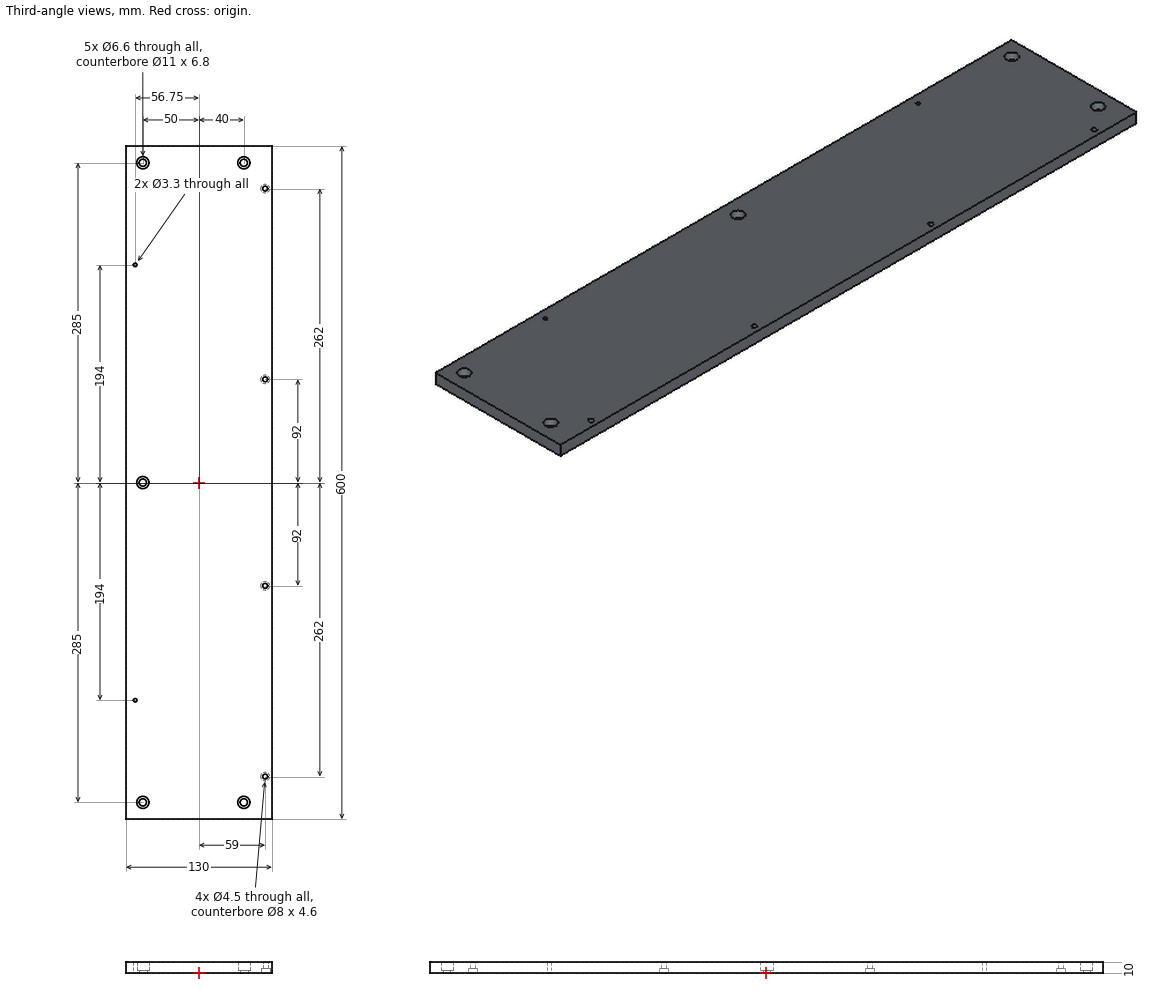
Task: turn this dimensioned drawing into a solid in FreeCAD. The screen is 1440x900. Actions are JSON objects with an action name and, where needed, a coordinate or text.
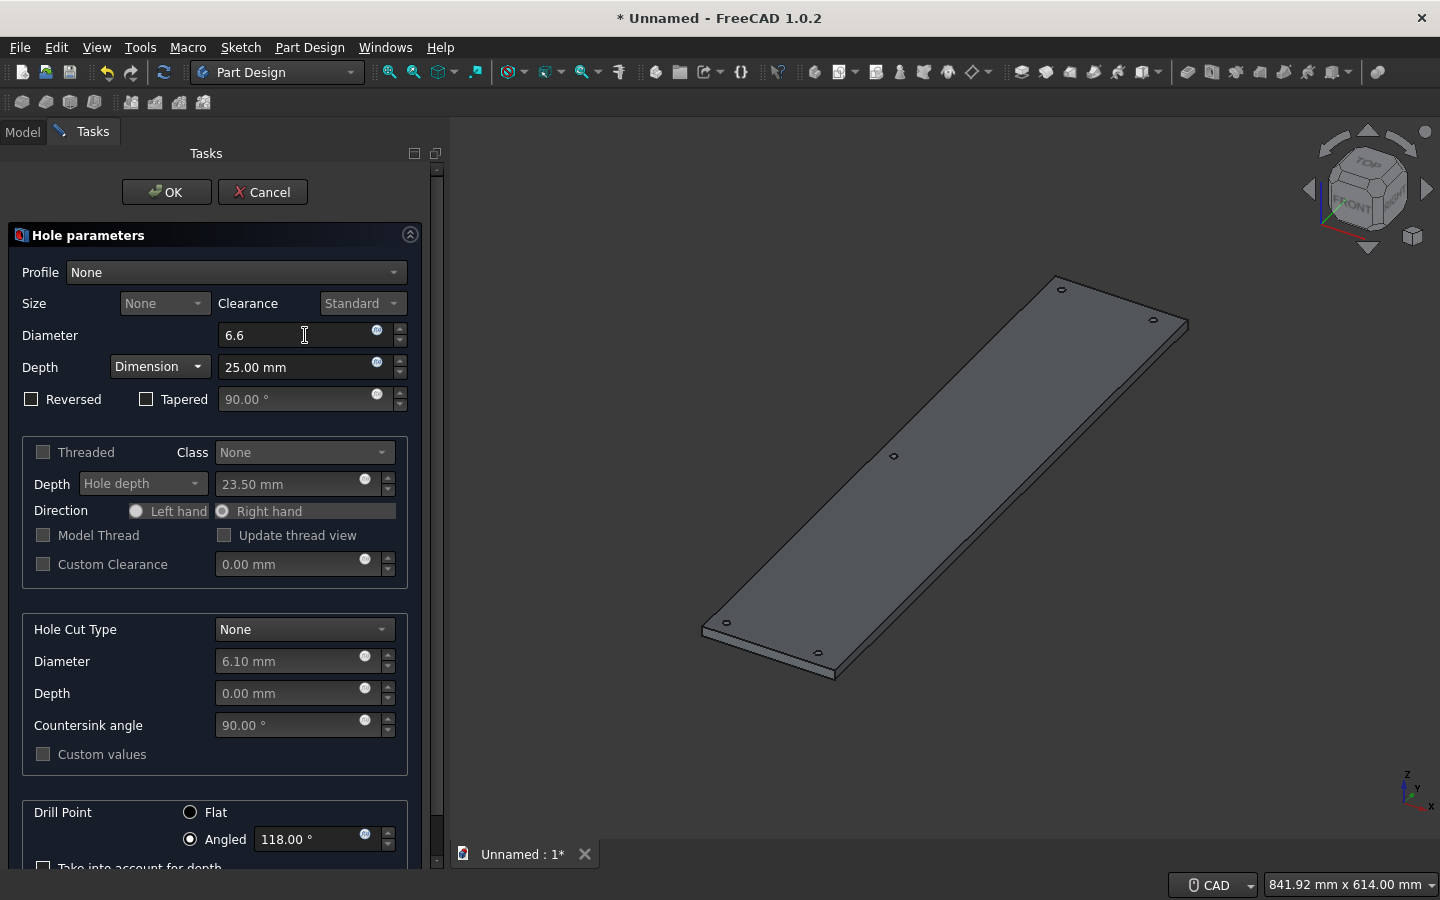
{"action": "left_click", "coordinate": [161, 366]}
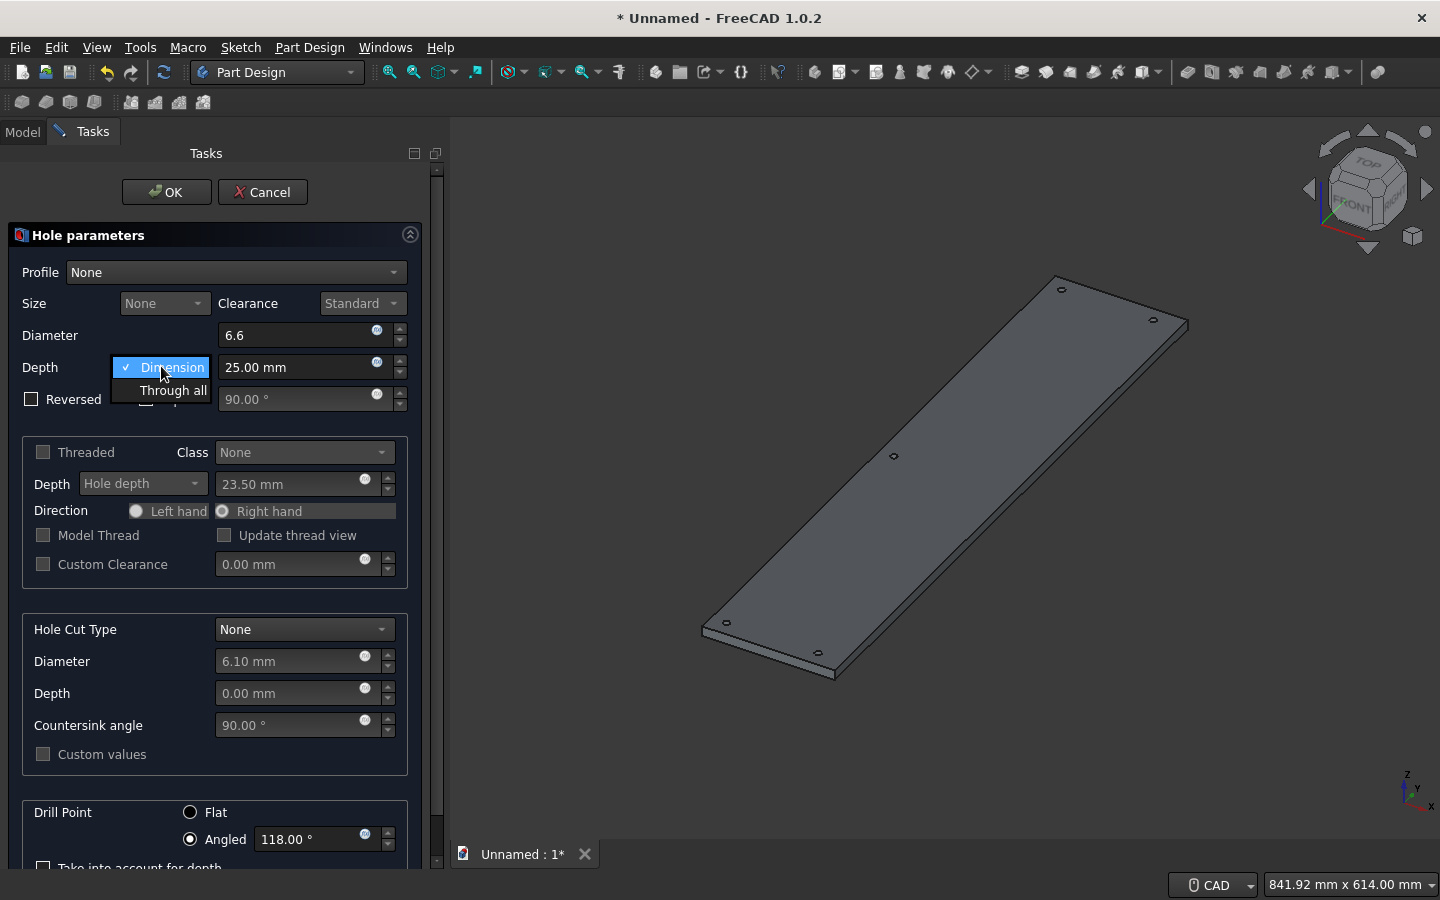
{"action": "left_click", "coordinate": [160, 390]}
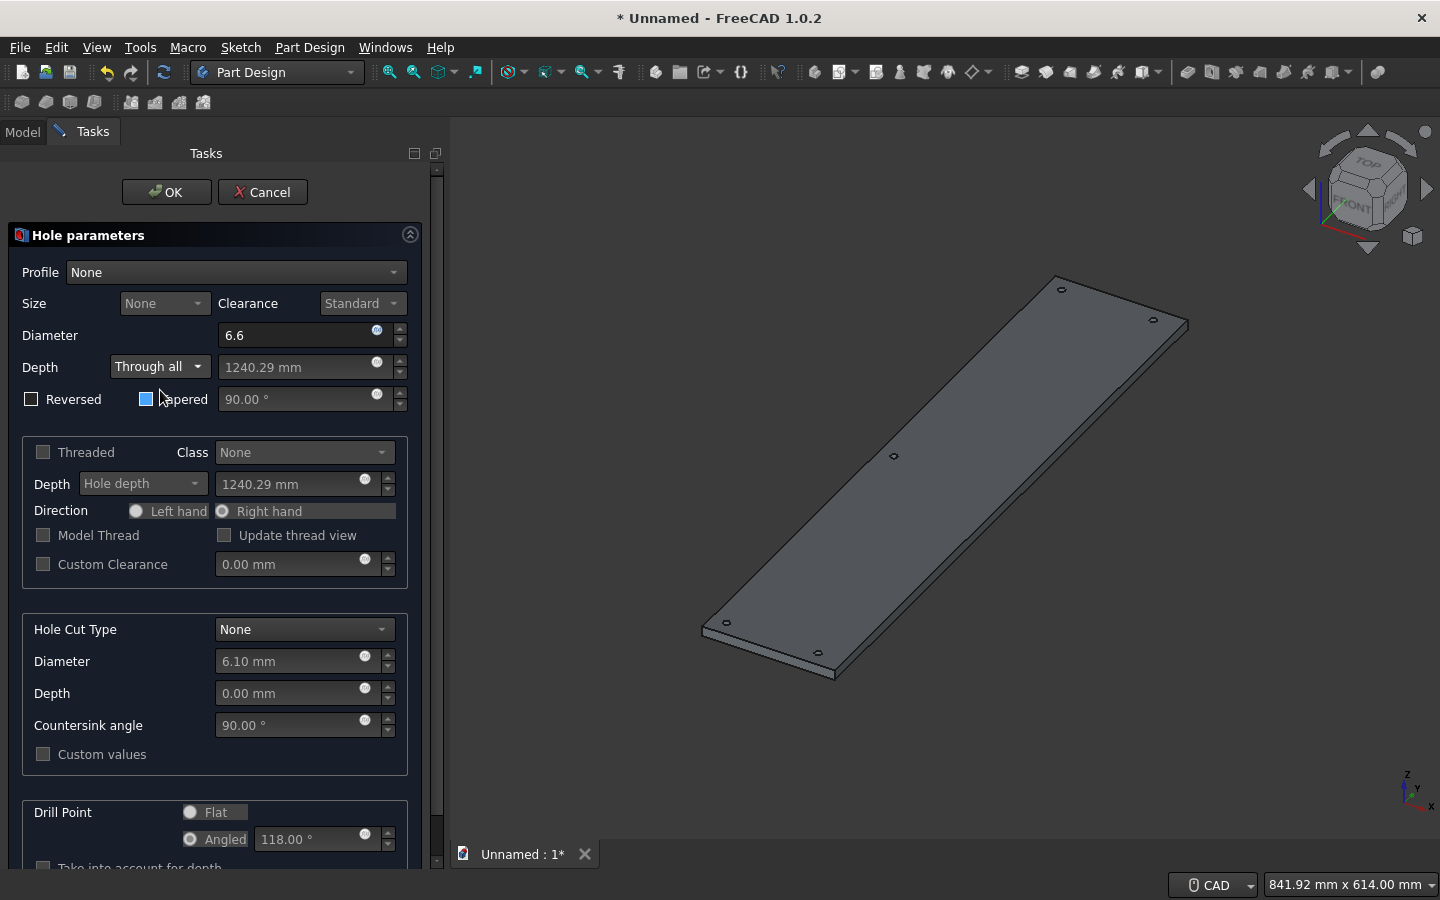
{"action": "left_click", "coordinate": [306, 630]}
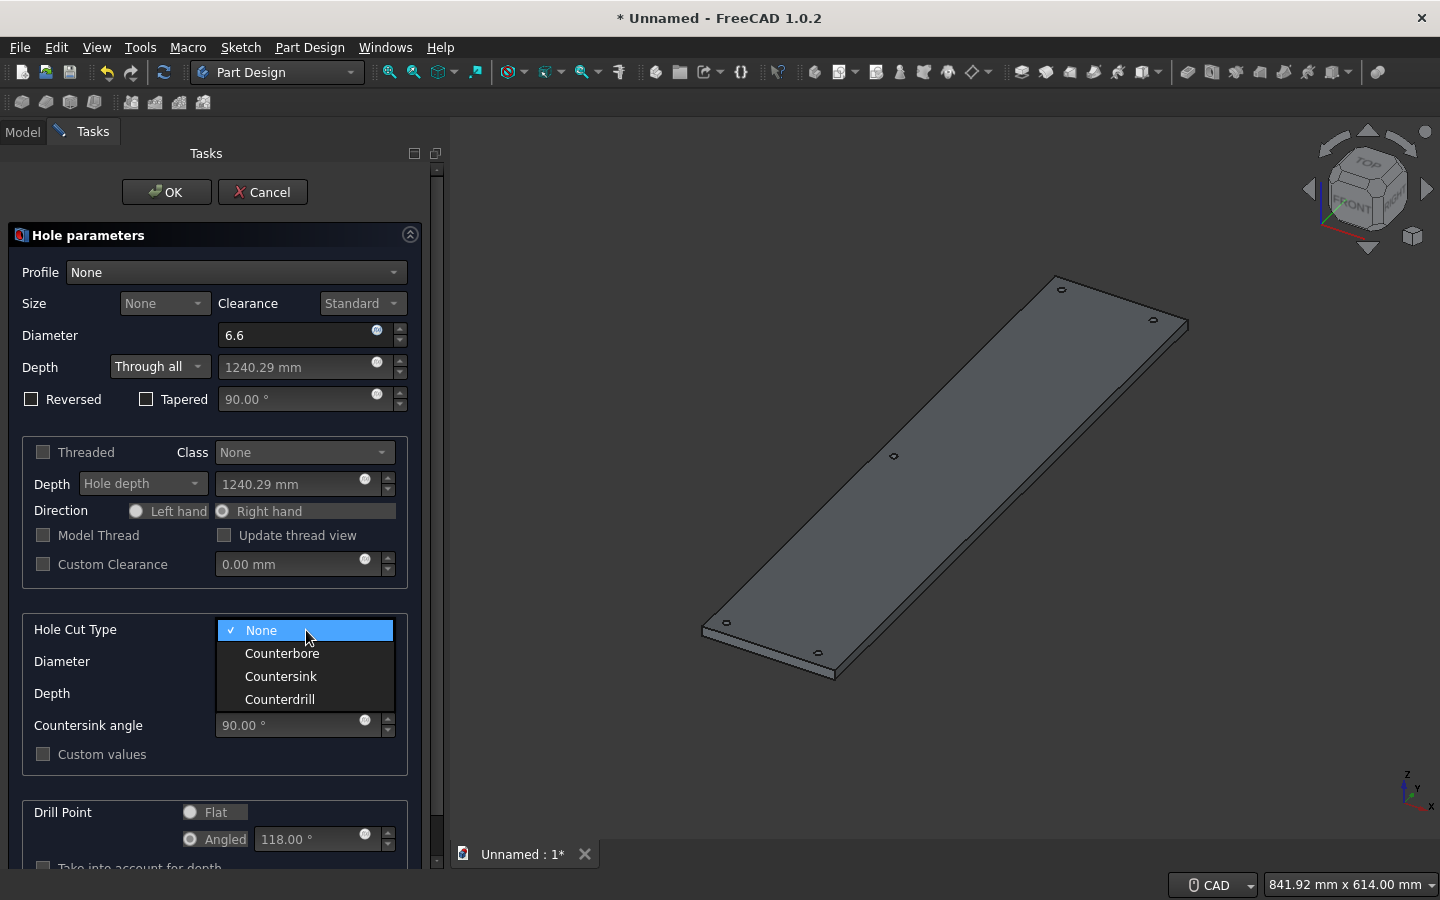
{"action": "left_click", "coordinate": [304, 654]}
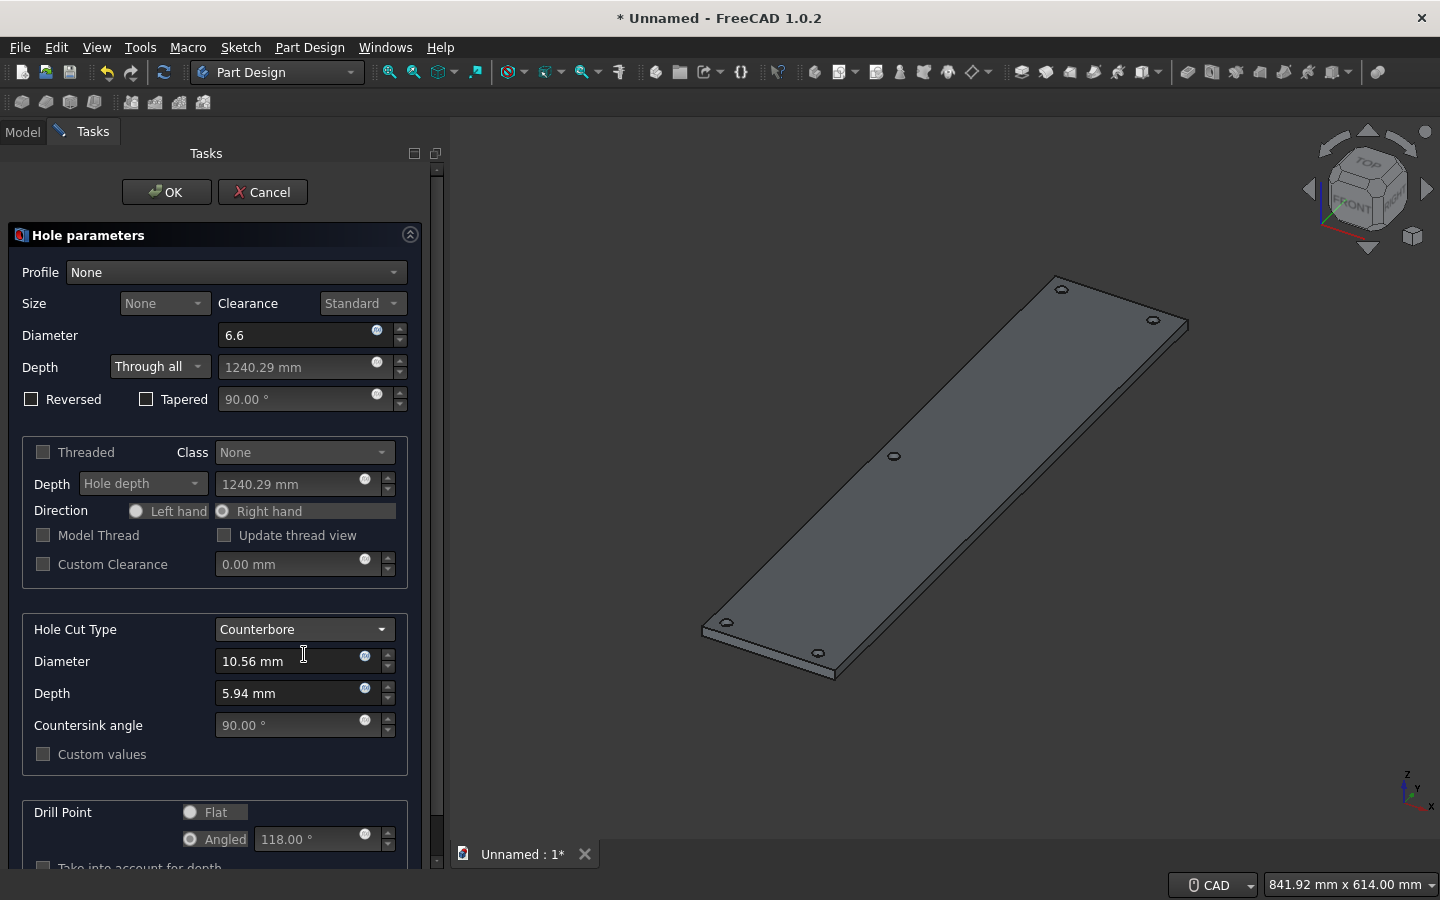
{"action": "triple_click", "coordinate": [298, 661]}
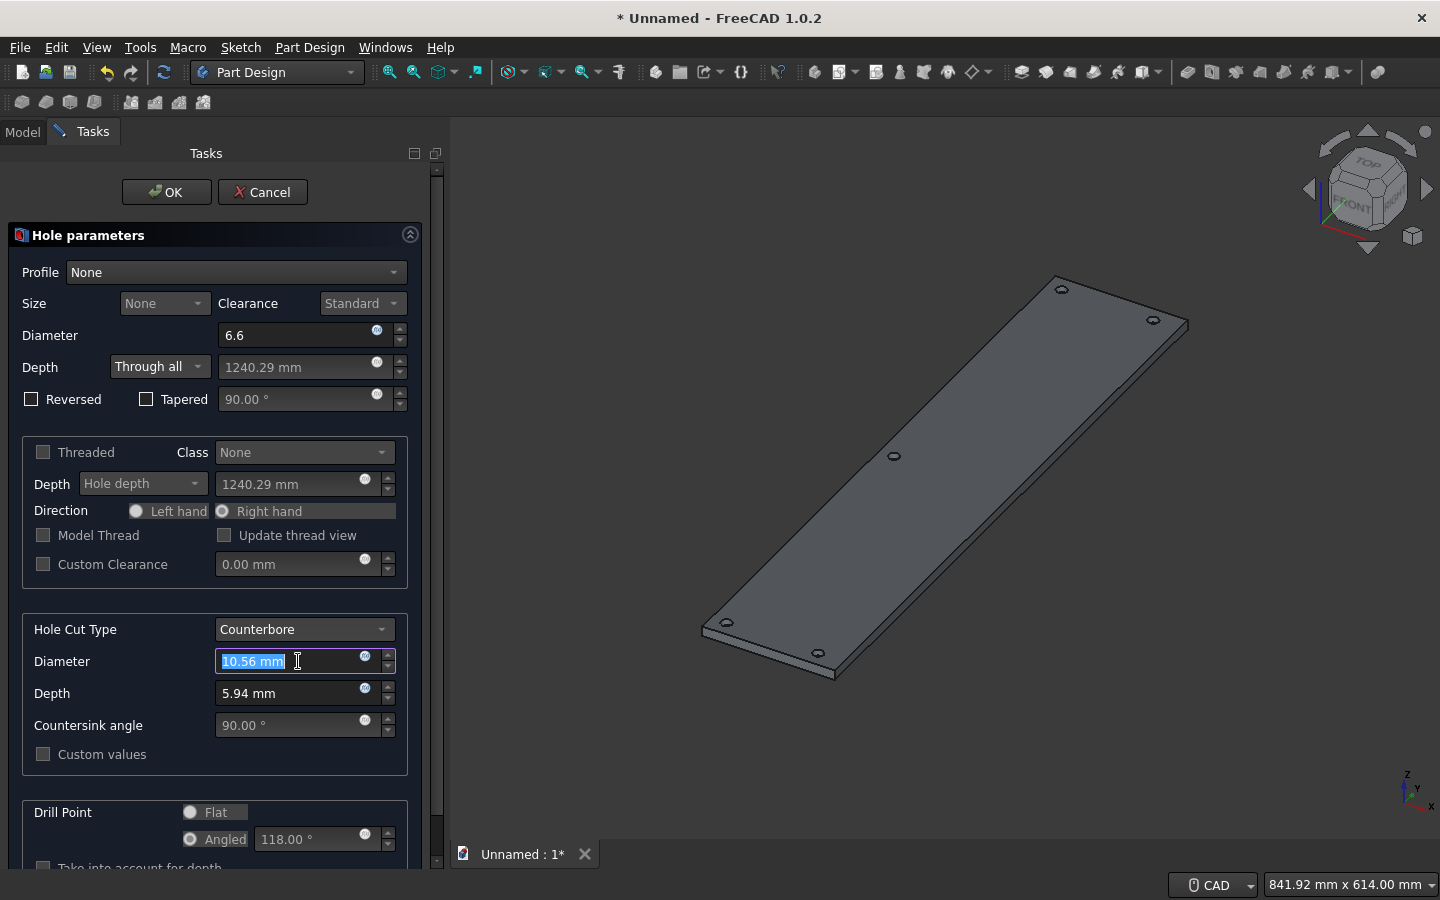
{"action": "type", "text": "11"}
{"action": "key", "text": "Tab"}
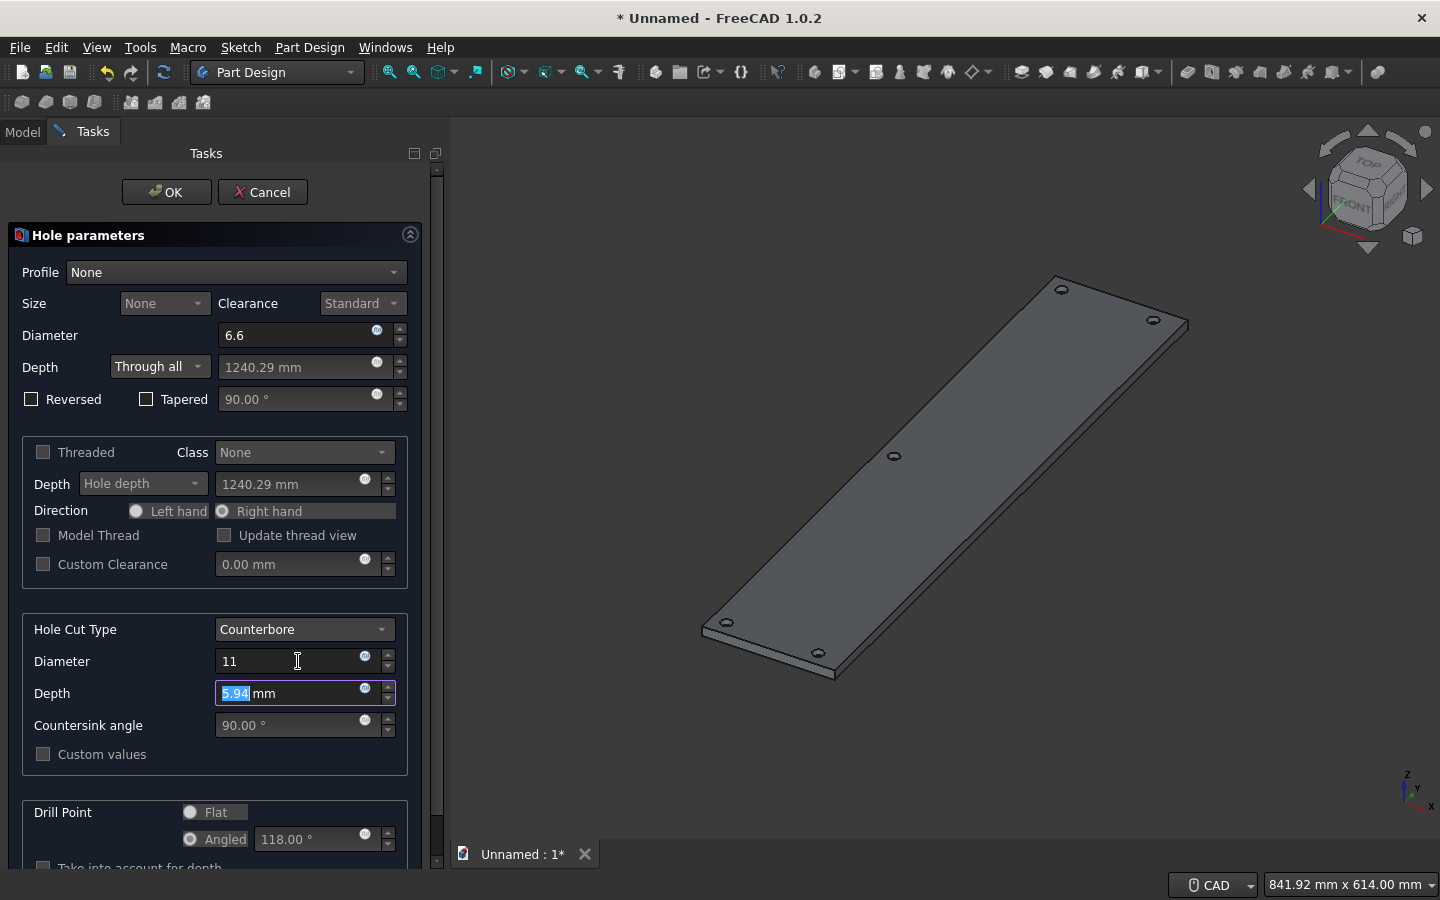
{"action": "type", "text": "6.8"}
{"action": "key", "text": "Tab"}